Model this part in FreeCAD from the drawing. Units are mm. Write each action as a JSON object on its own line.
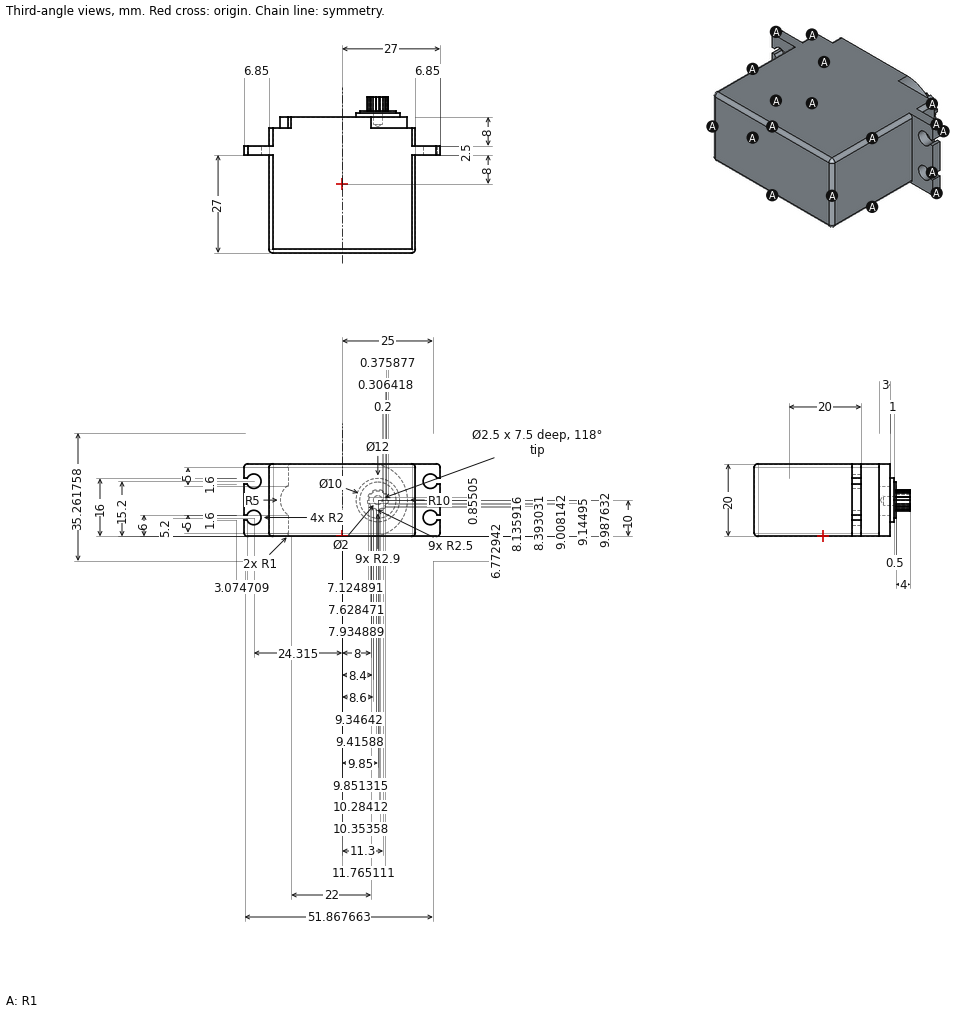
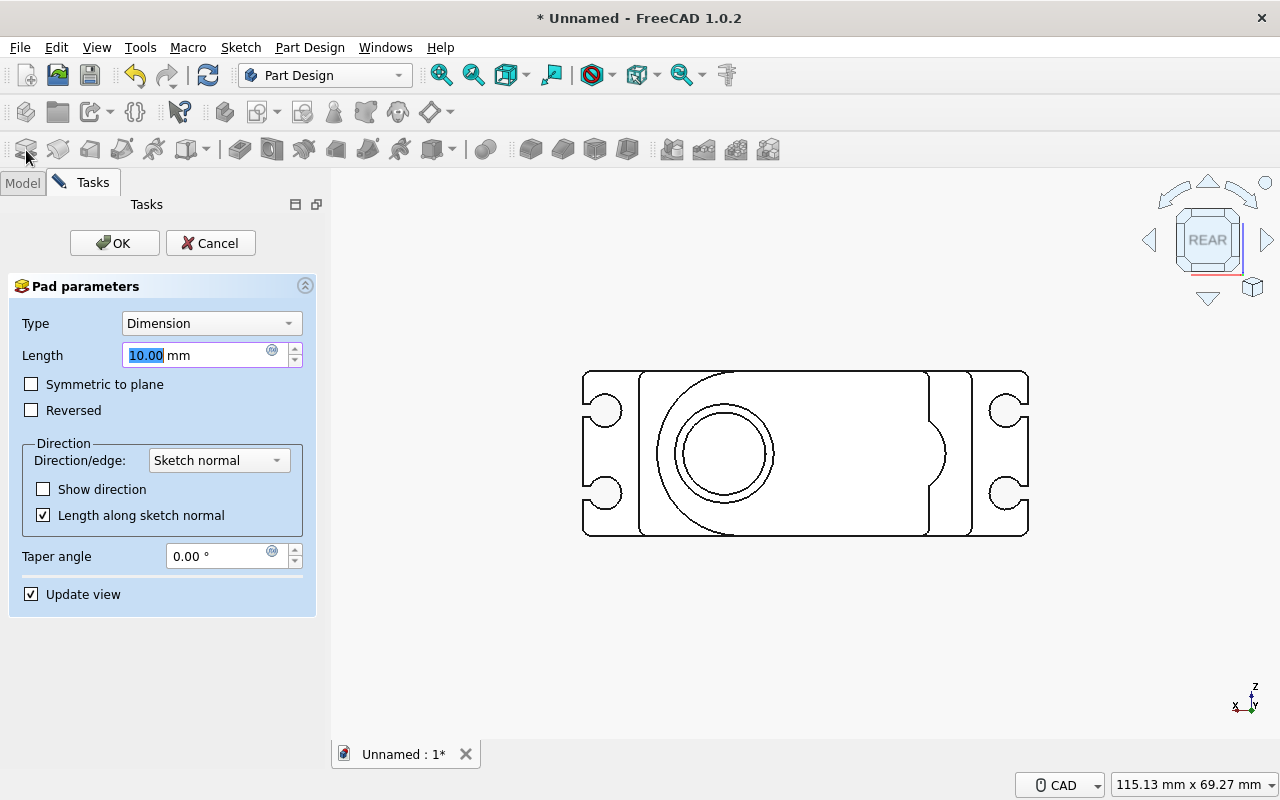
{"action": "type", "text": "0.5"}
{"action": "key", "text": "Tab"}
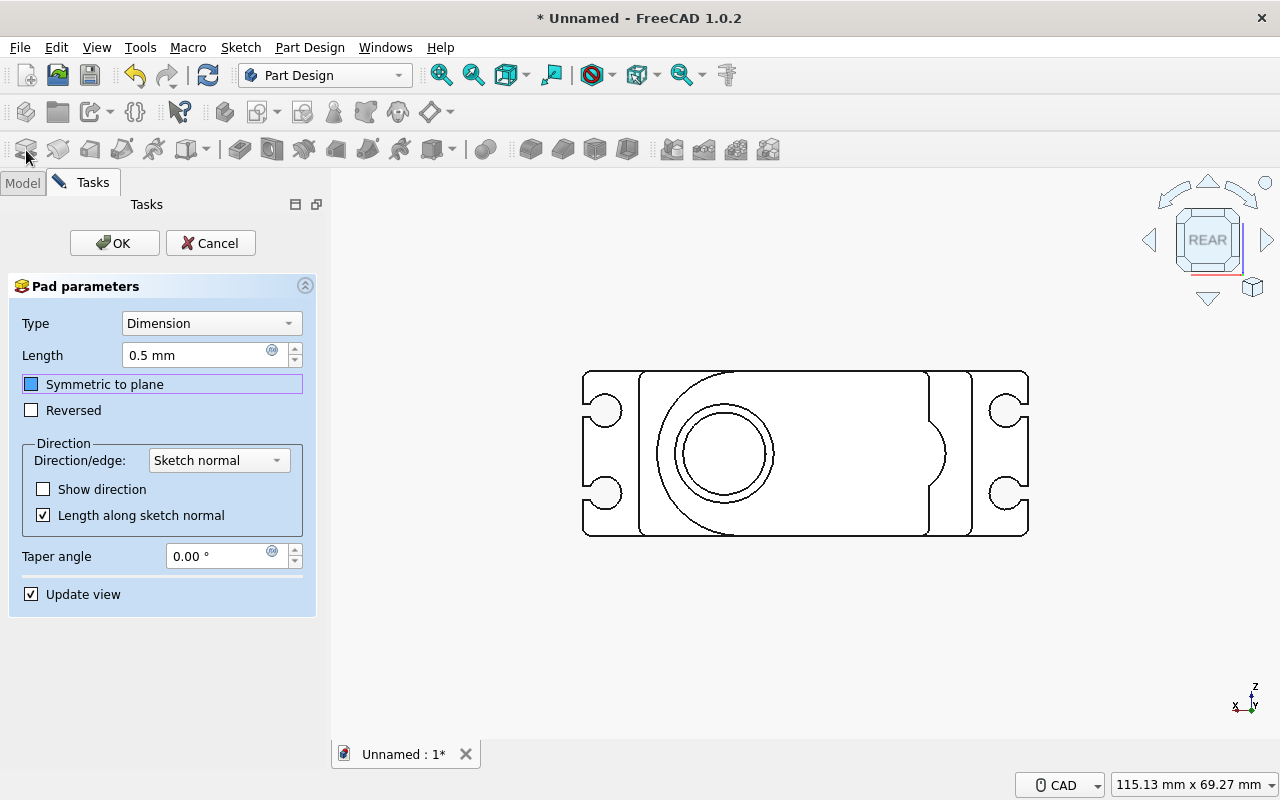
{"action": "left_click", "coordinate": [115, 243]}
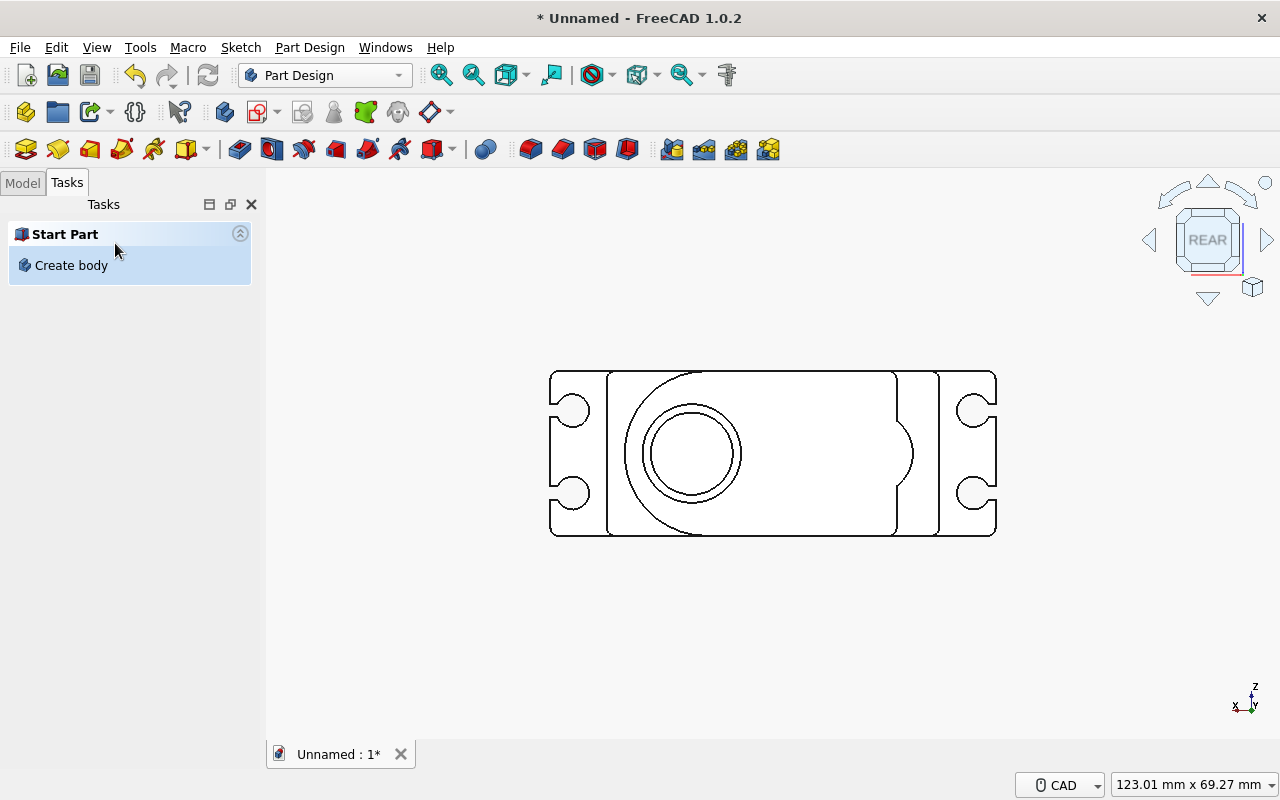
{"action": "left_click", "coordinate": [442, 76]}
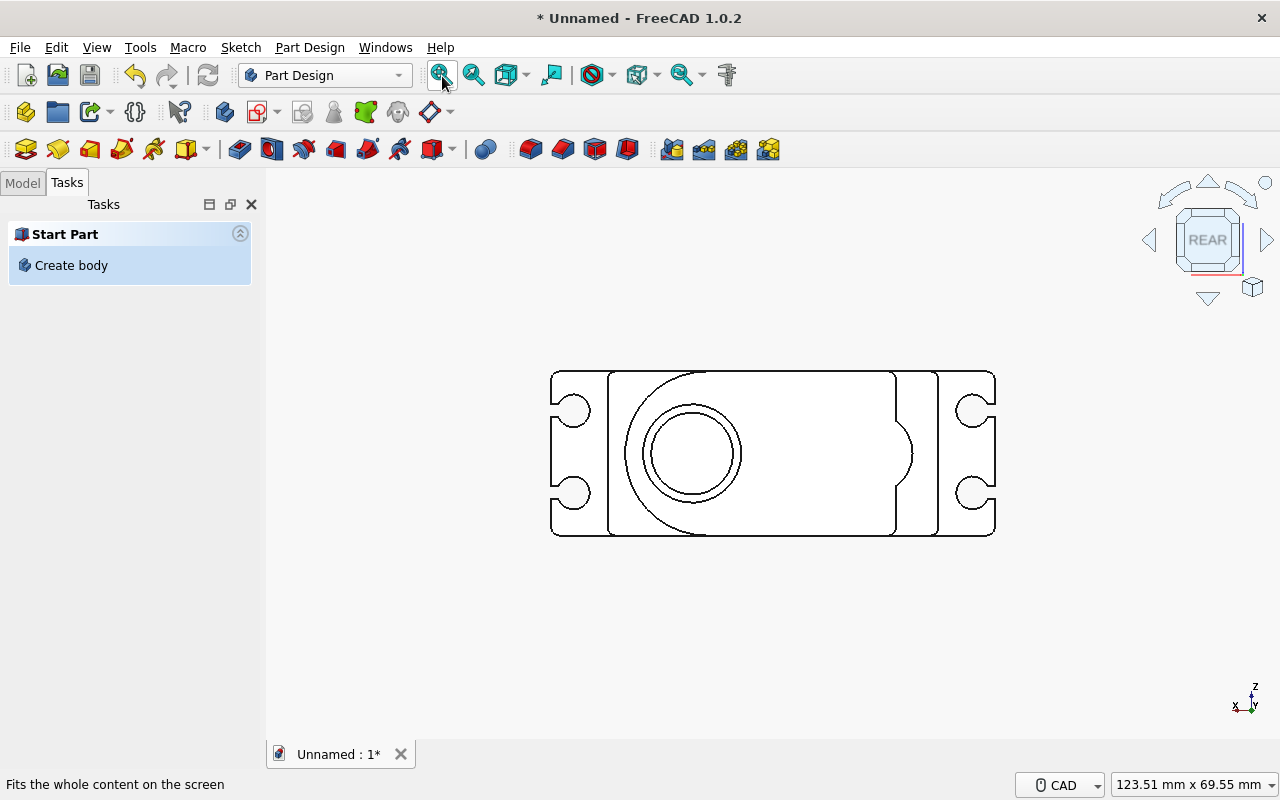
{"action": "left_click", "coordinate": [692, 453]}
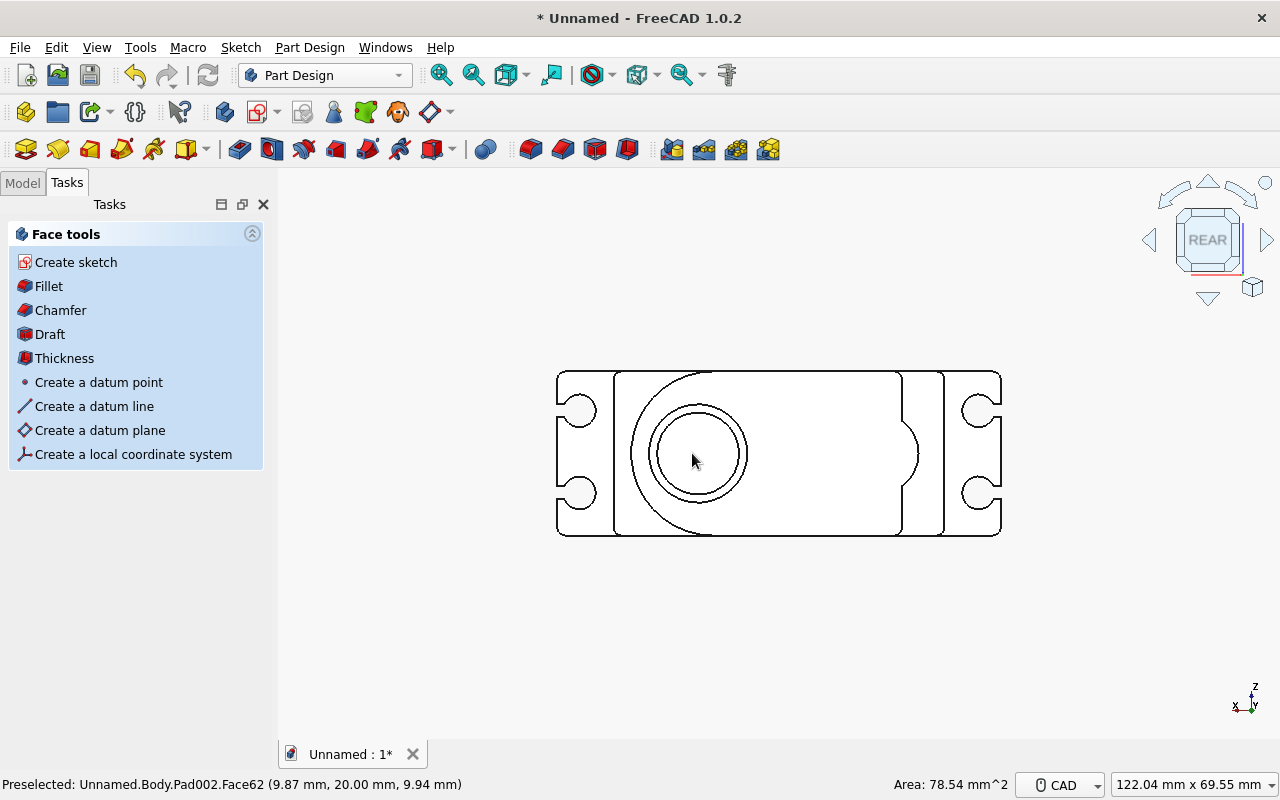
{"action": "left_click", "coordinate": [258, 112]}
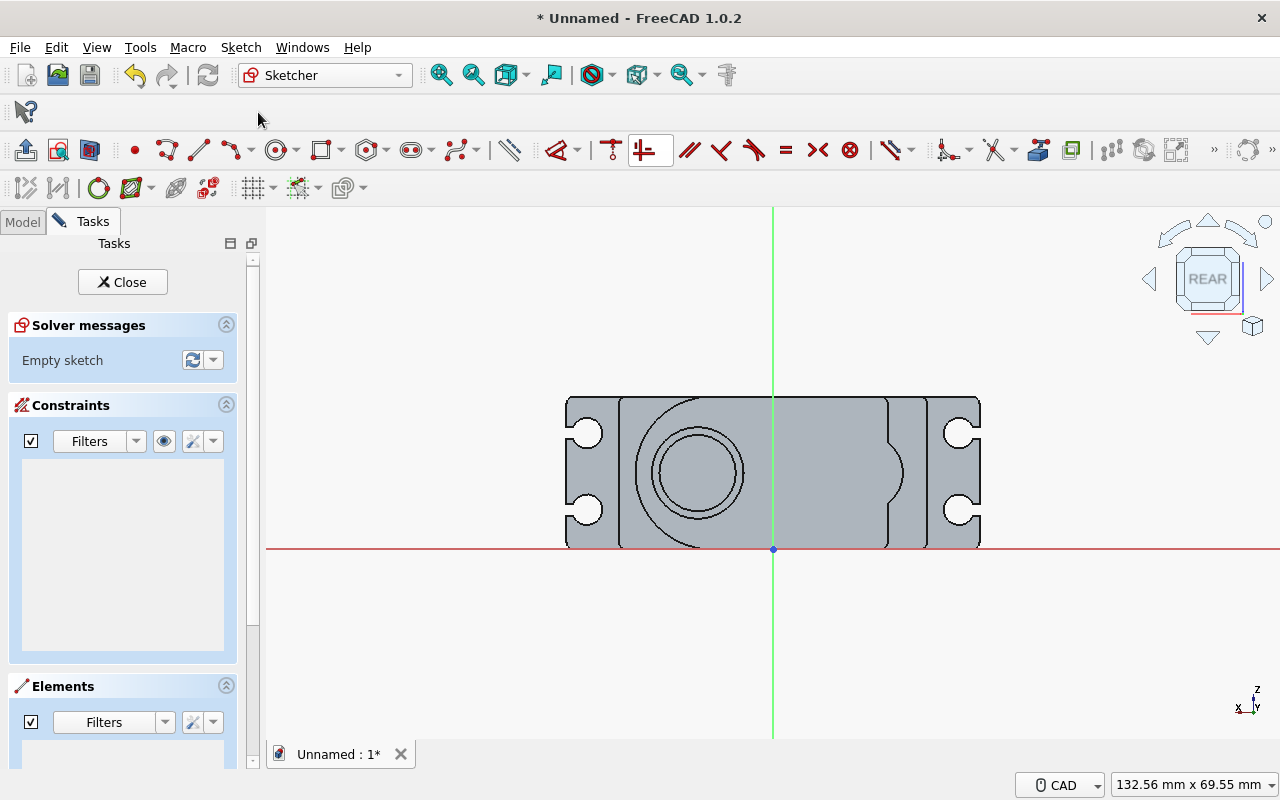
{"action": "scroll", "coordinate": [733, 512], "scroll_direction": "up", "scroll_amount": 6}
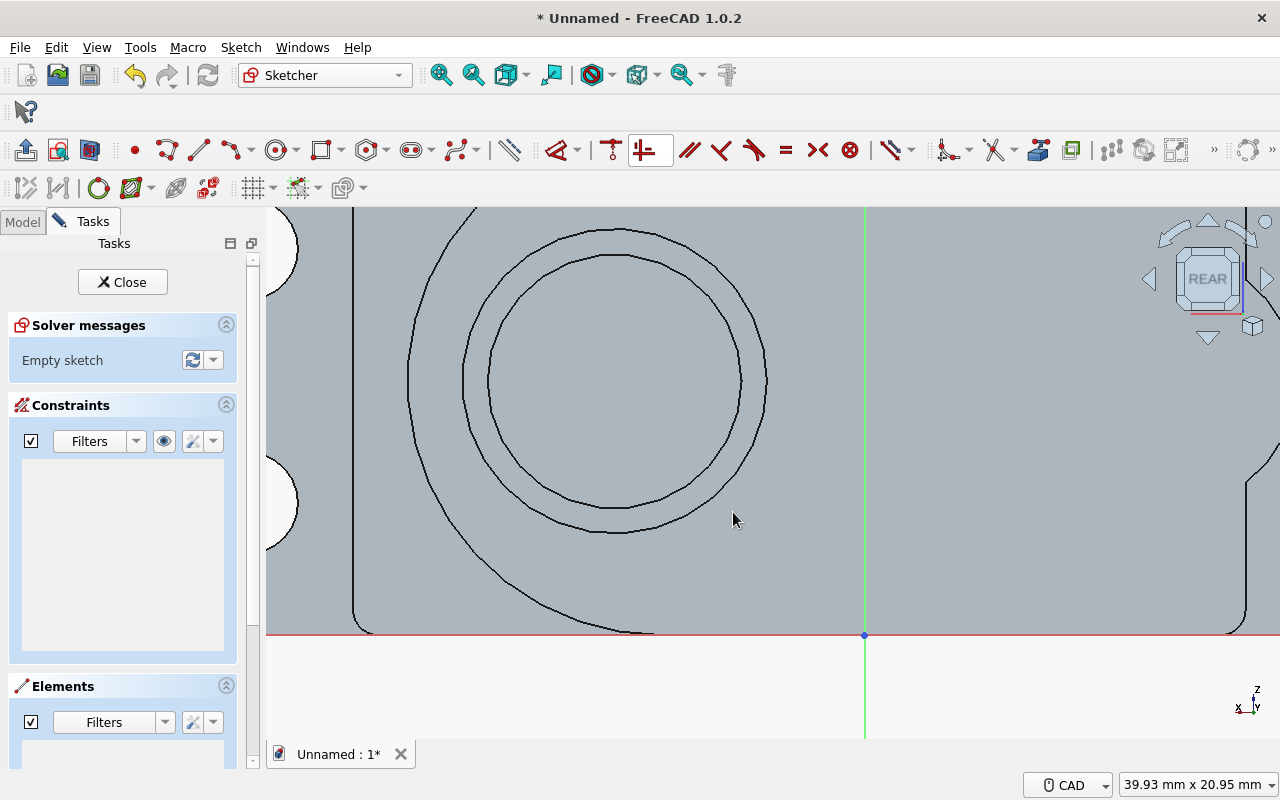
{"action": "left_click", "coordinate": [200, 150]}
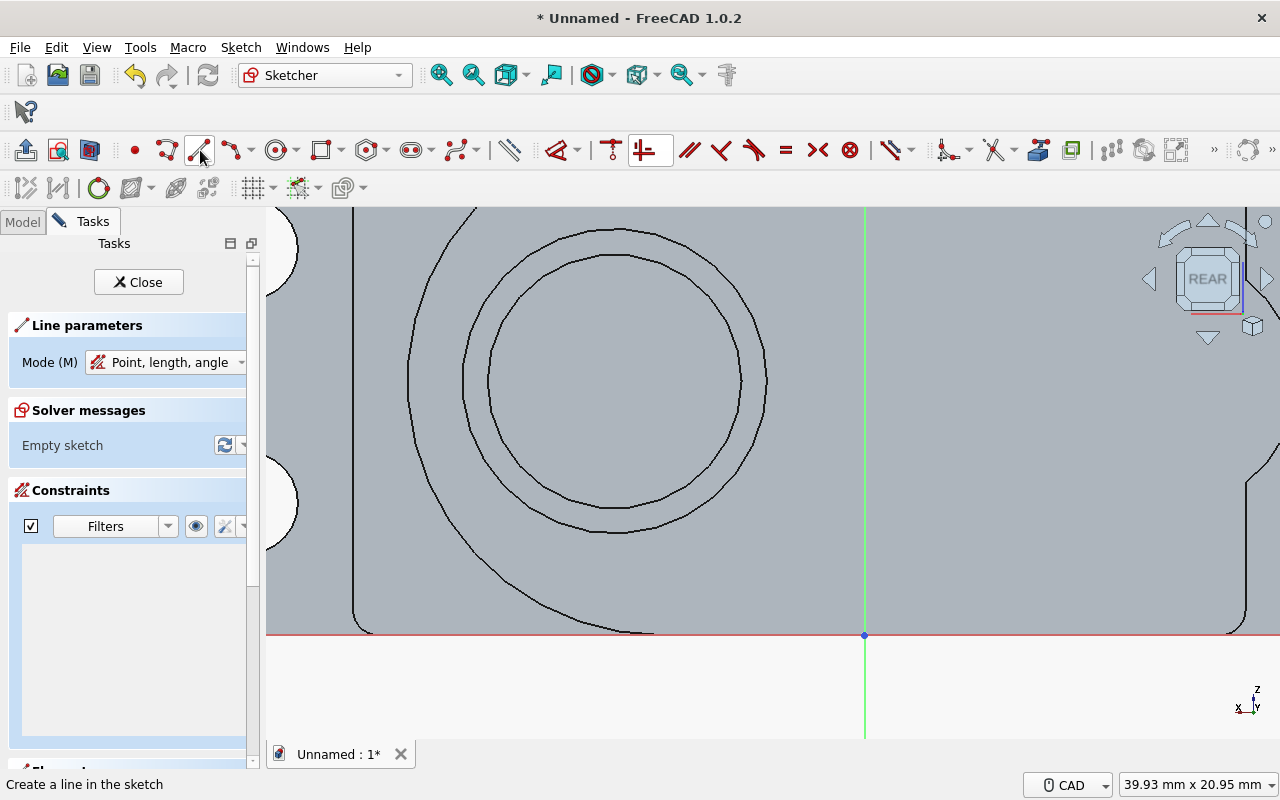
{"action": "left_click", "coordinate": [604, 444]}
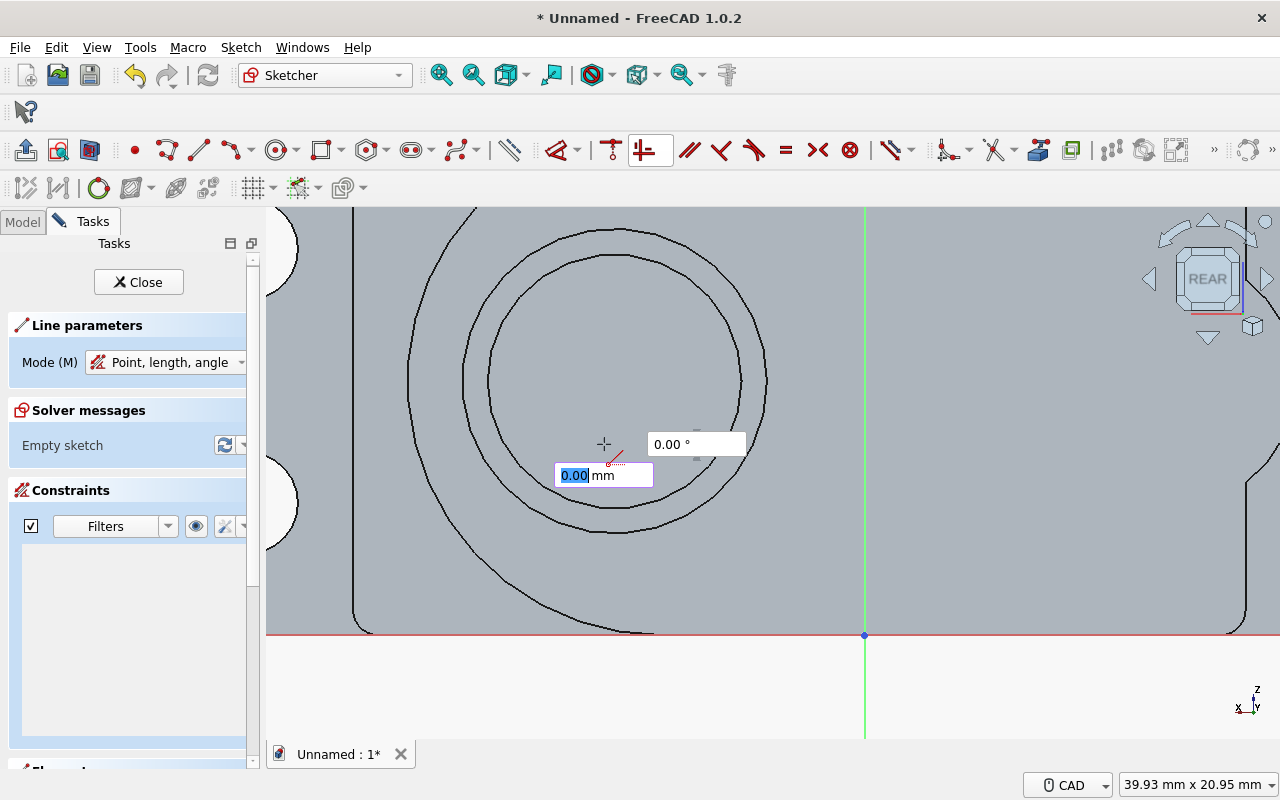
{"action": "scroll", "coordinate": [602, 454], "scroll_direction": "up", "scroll_amount": 3}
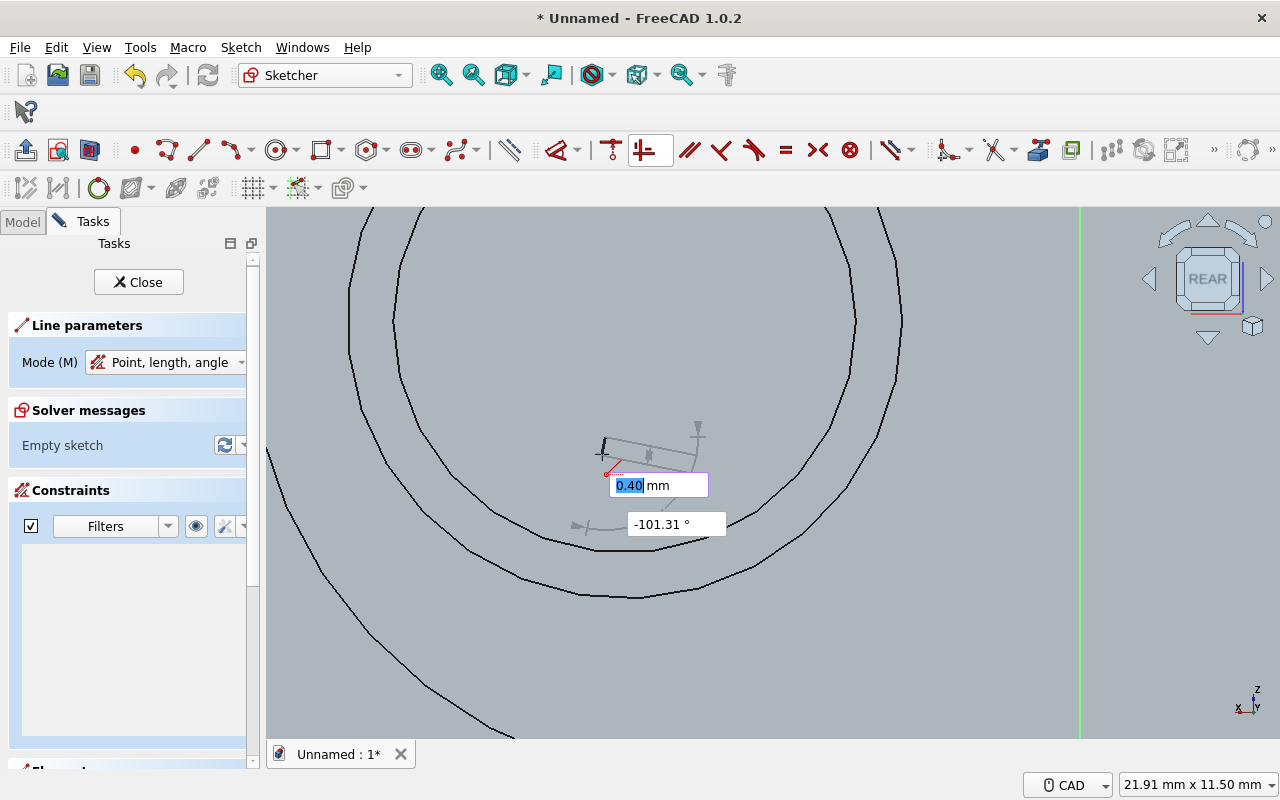
{"action": "left_click", "coordinate": [601, 453]}